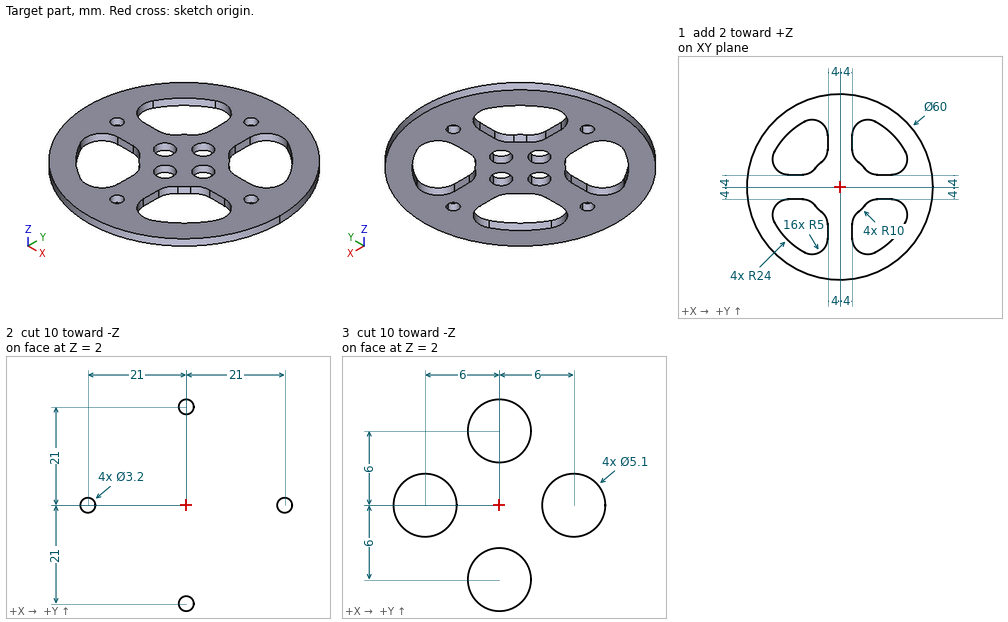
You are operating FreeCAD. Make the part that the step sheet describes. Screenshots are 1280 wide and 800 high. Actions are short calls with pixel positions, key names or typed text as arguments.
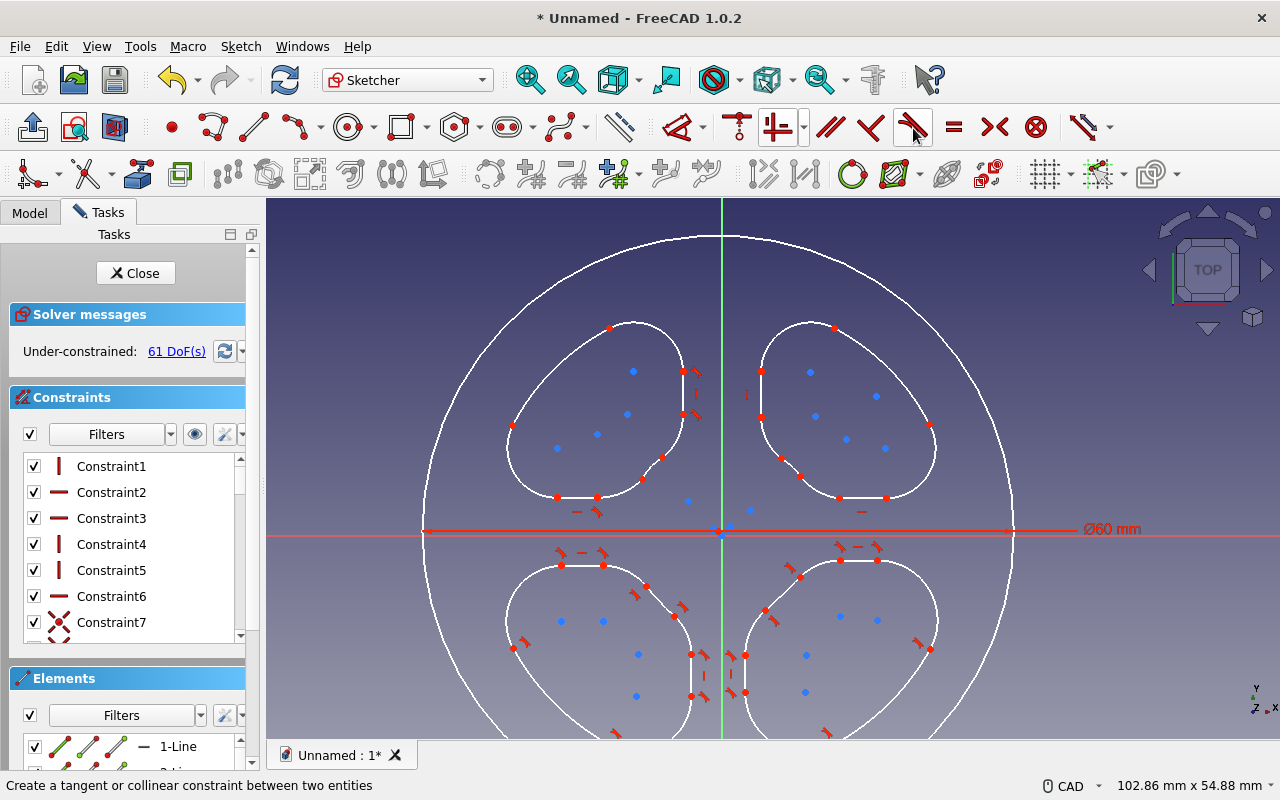
click(585, 498)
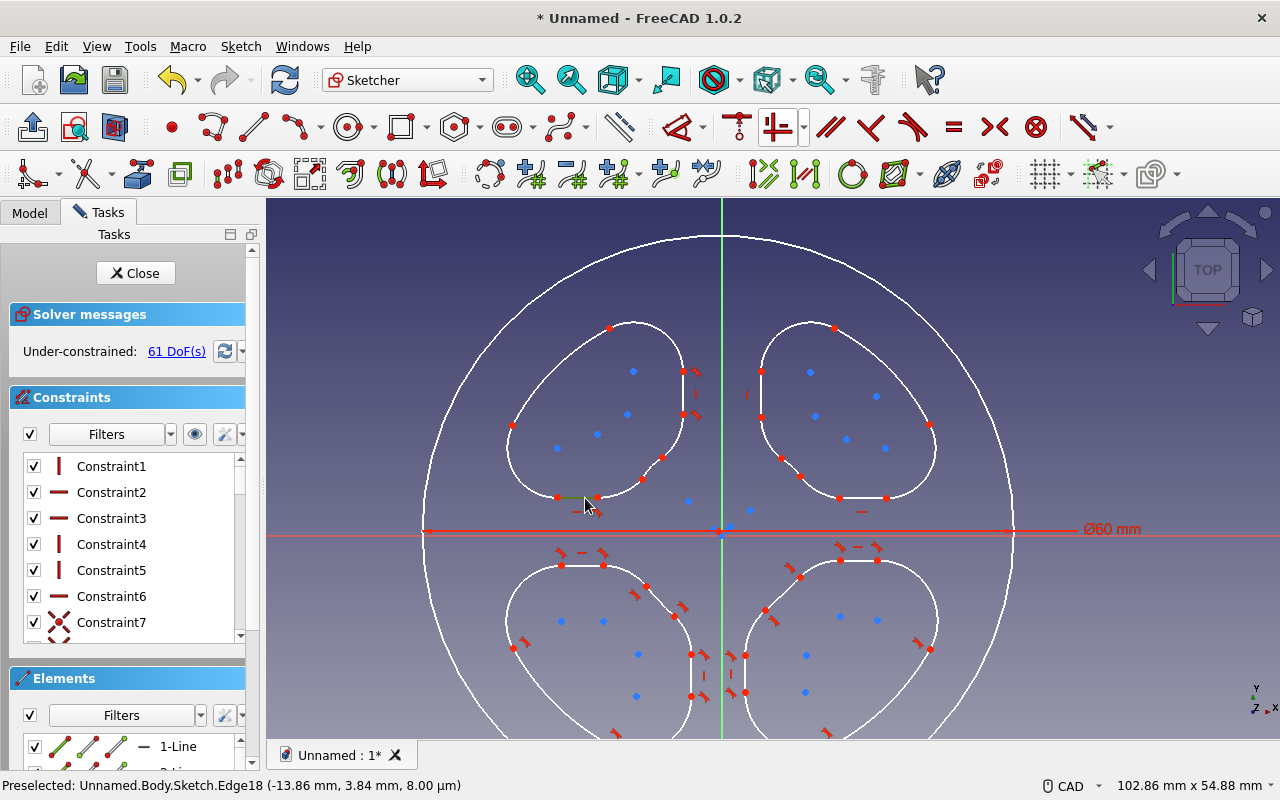
click(508, 455)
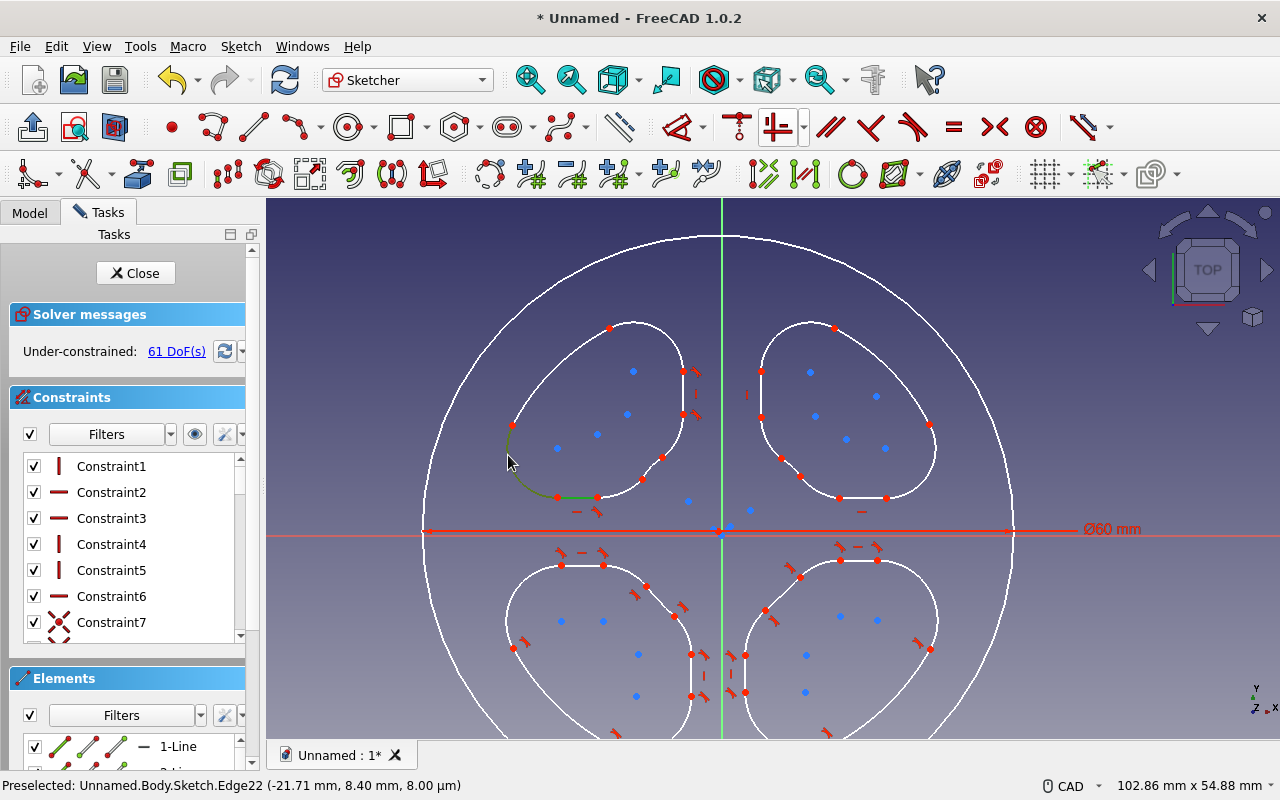
click(913, 128)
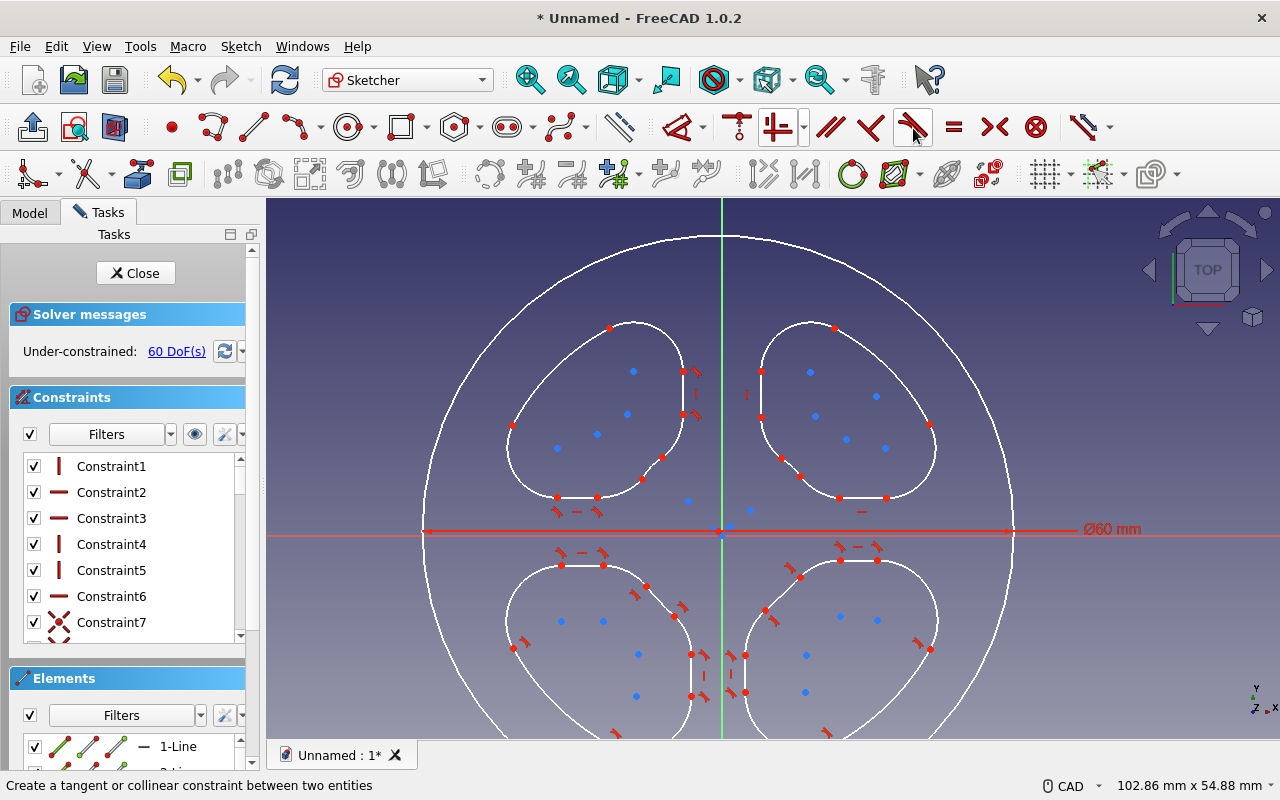
click(673, 447)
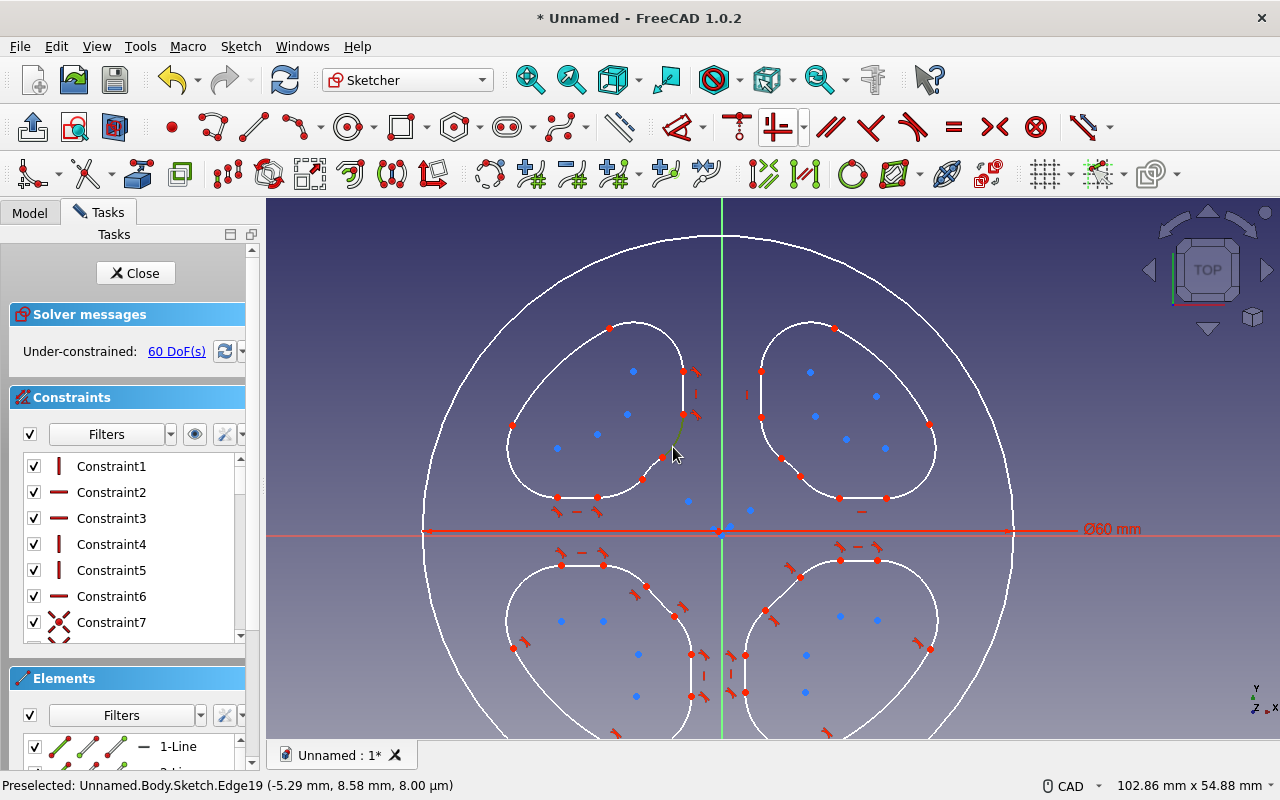
click(651, 467)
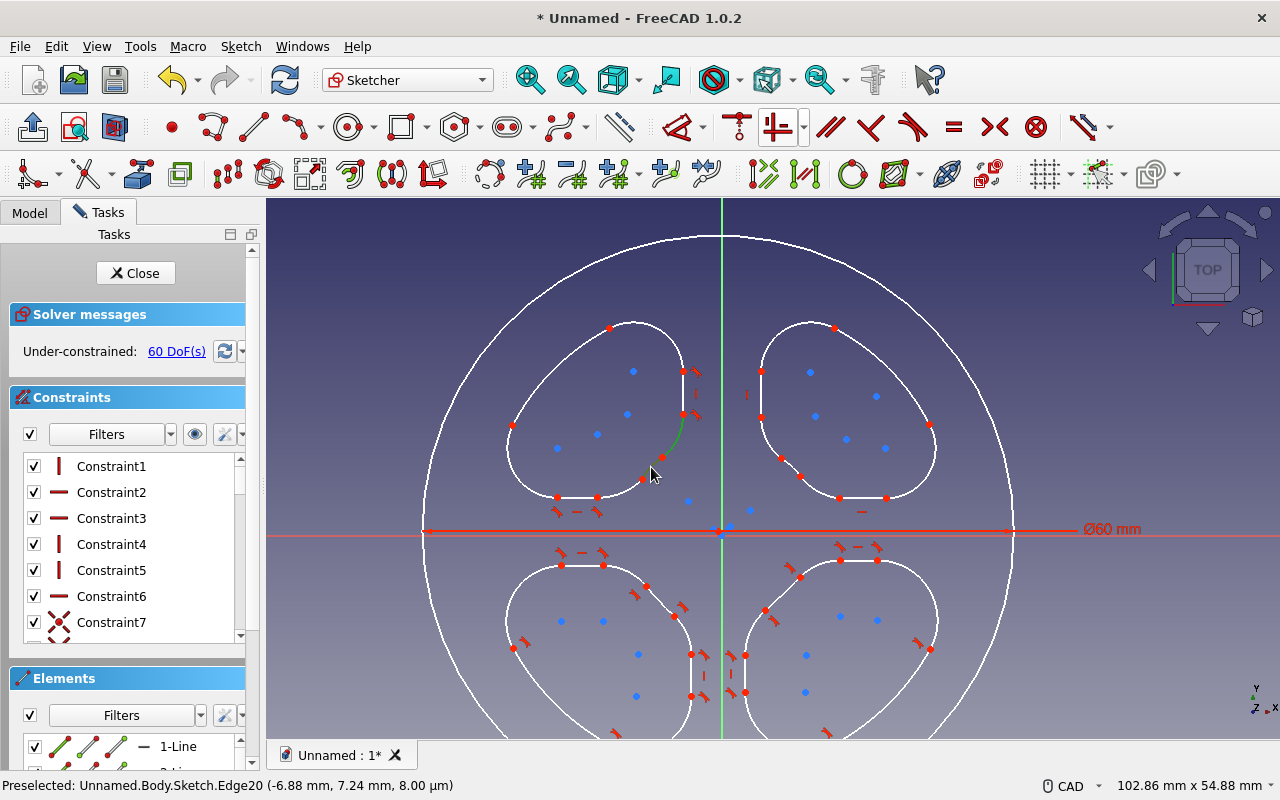
click(913, 128)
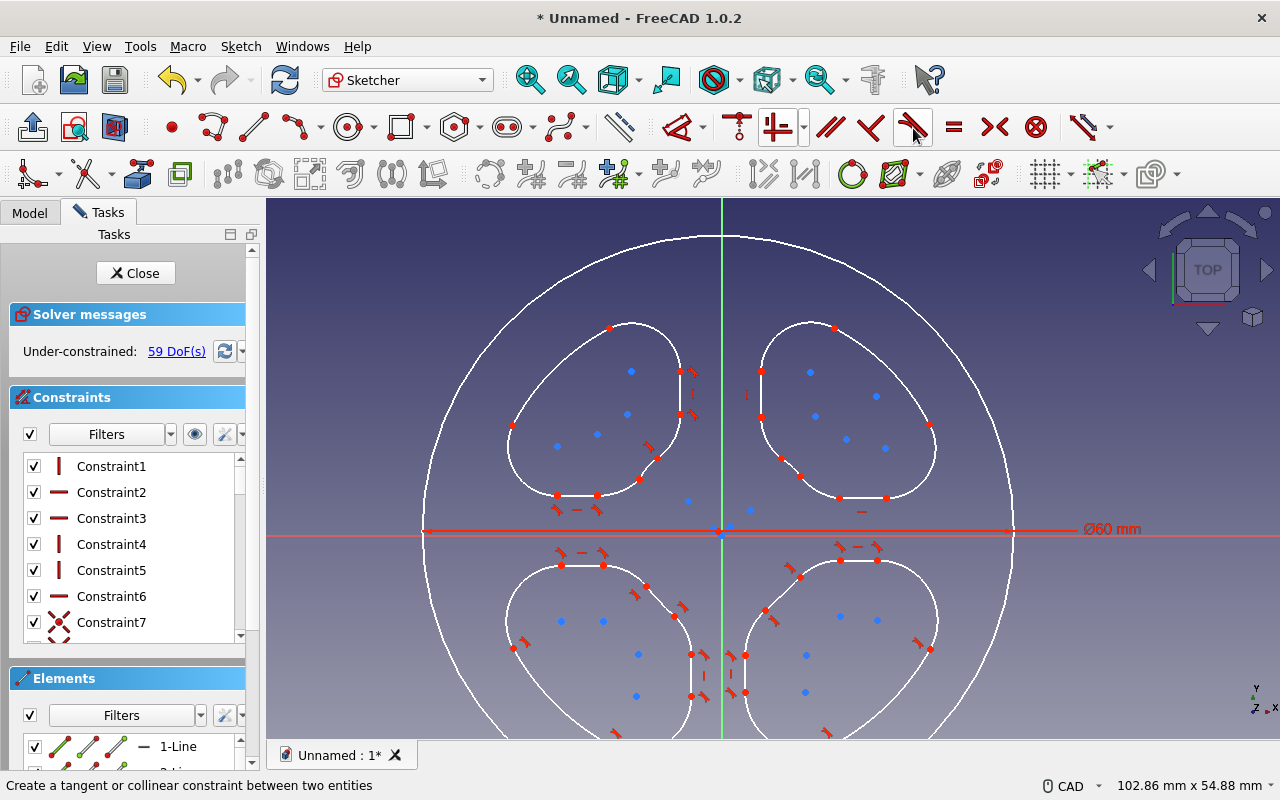
click(647, 467)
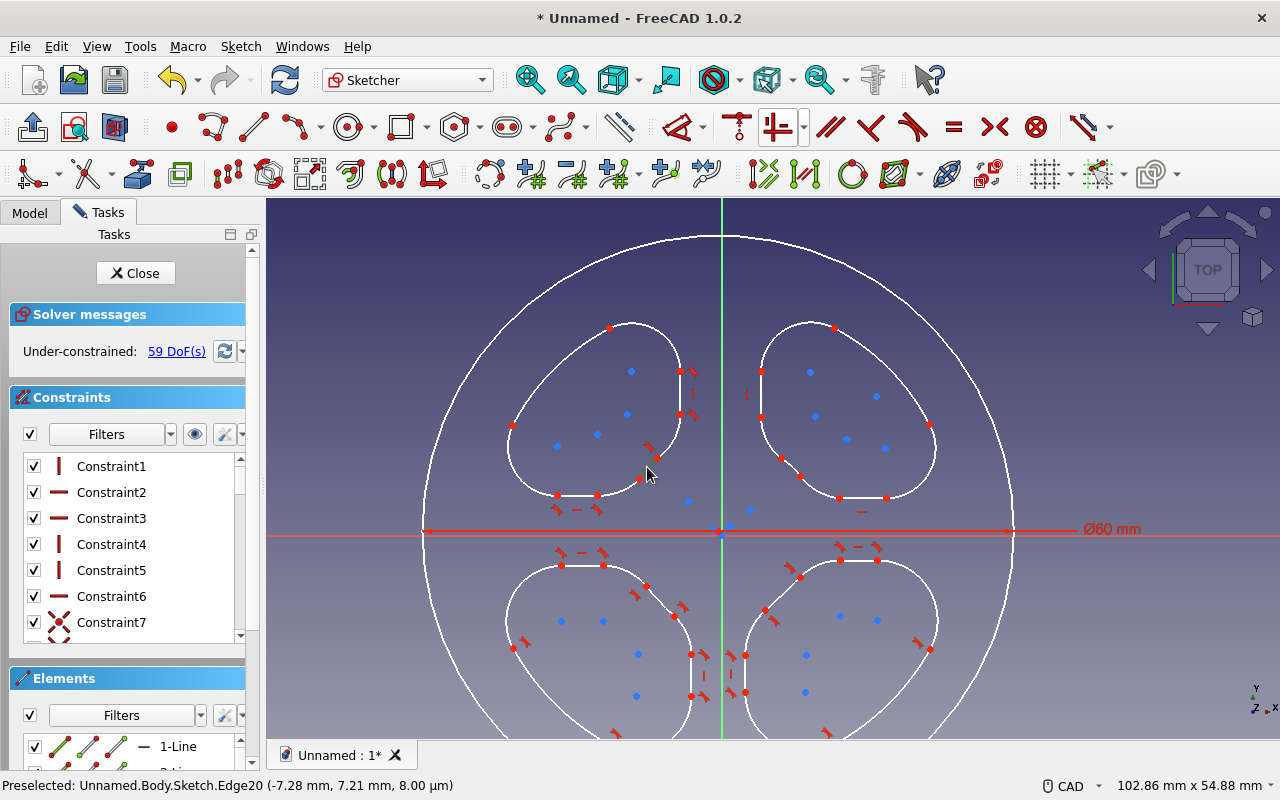
click(611, 494)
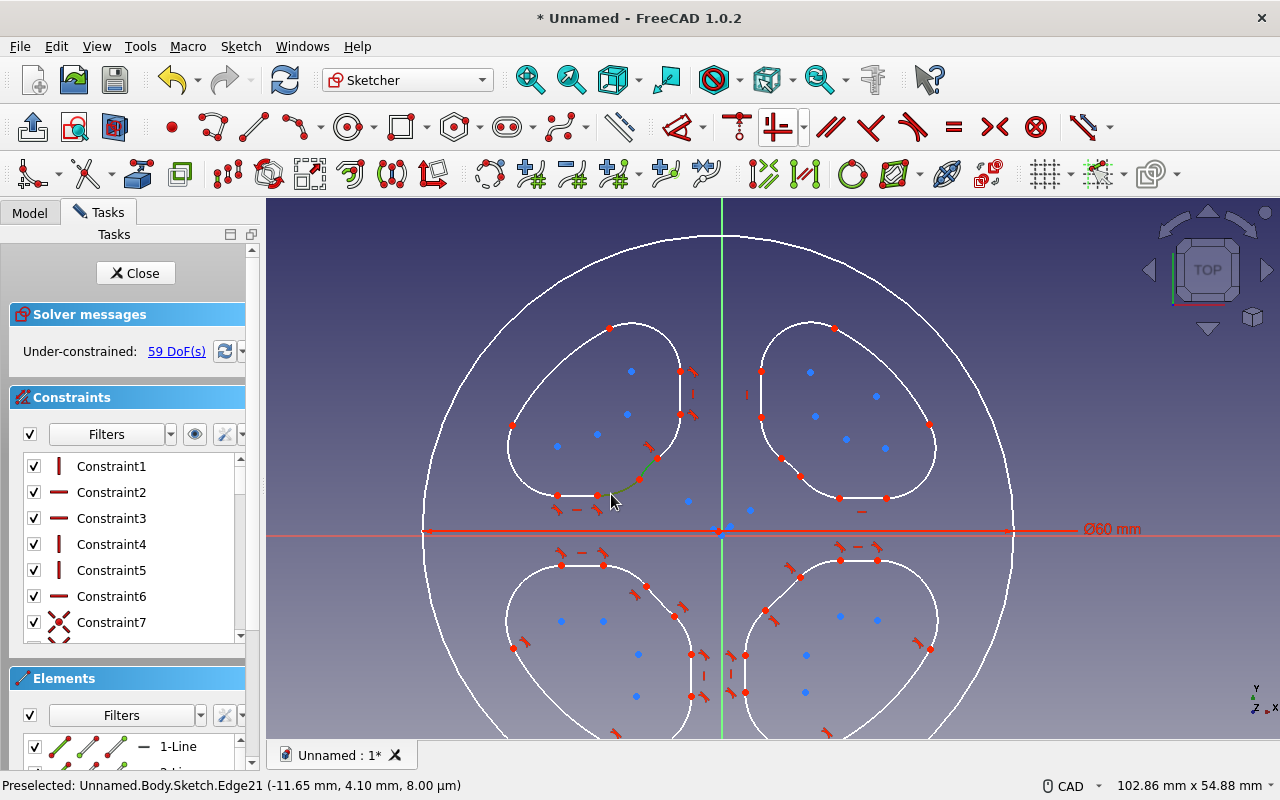
click(913, 128)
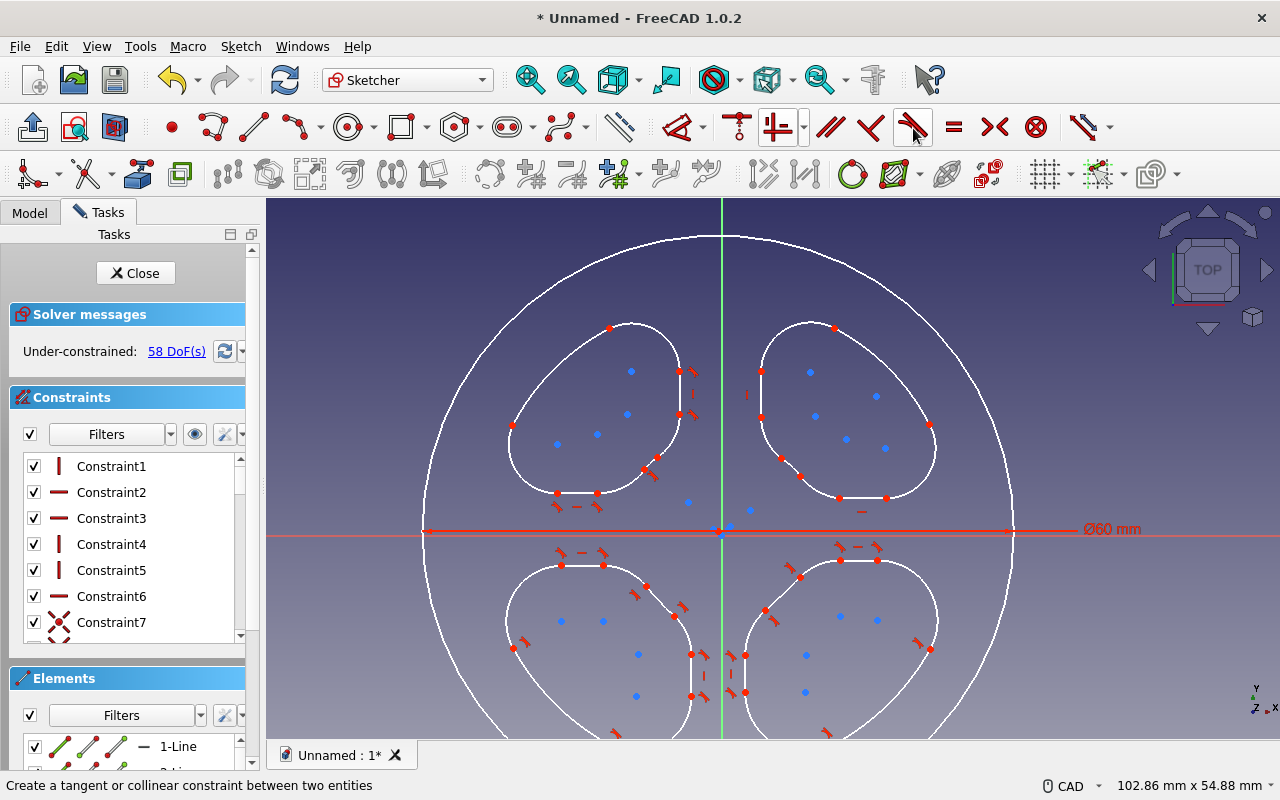
click(510, 453)